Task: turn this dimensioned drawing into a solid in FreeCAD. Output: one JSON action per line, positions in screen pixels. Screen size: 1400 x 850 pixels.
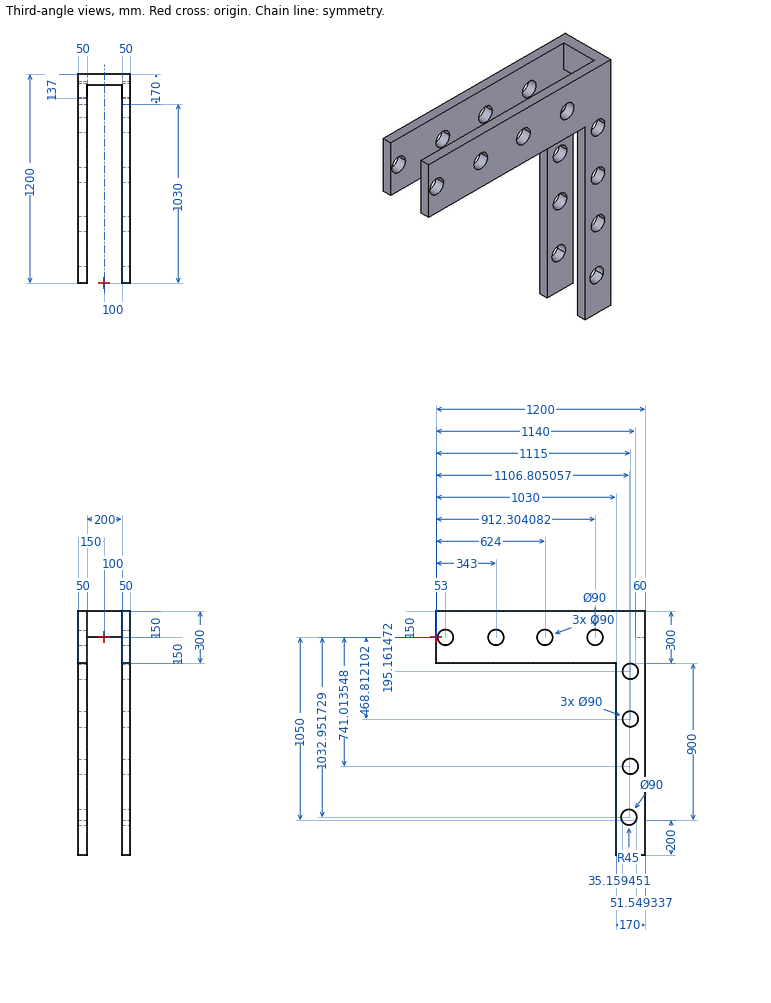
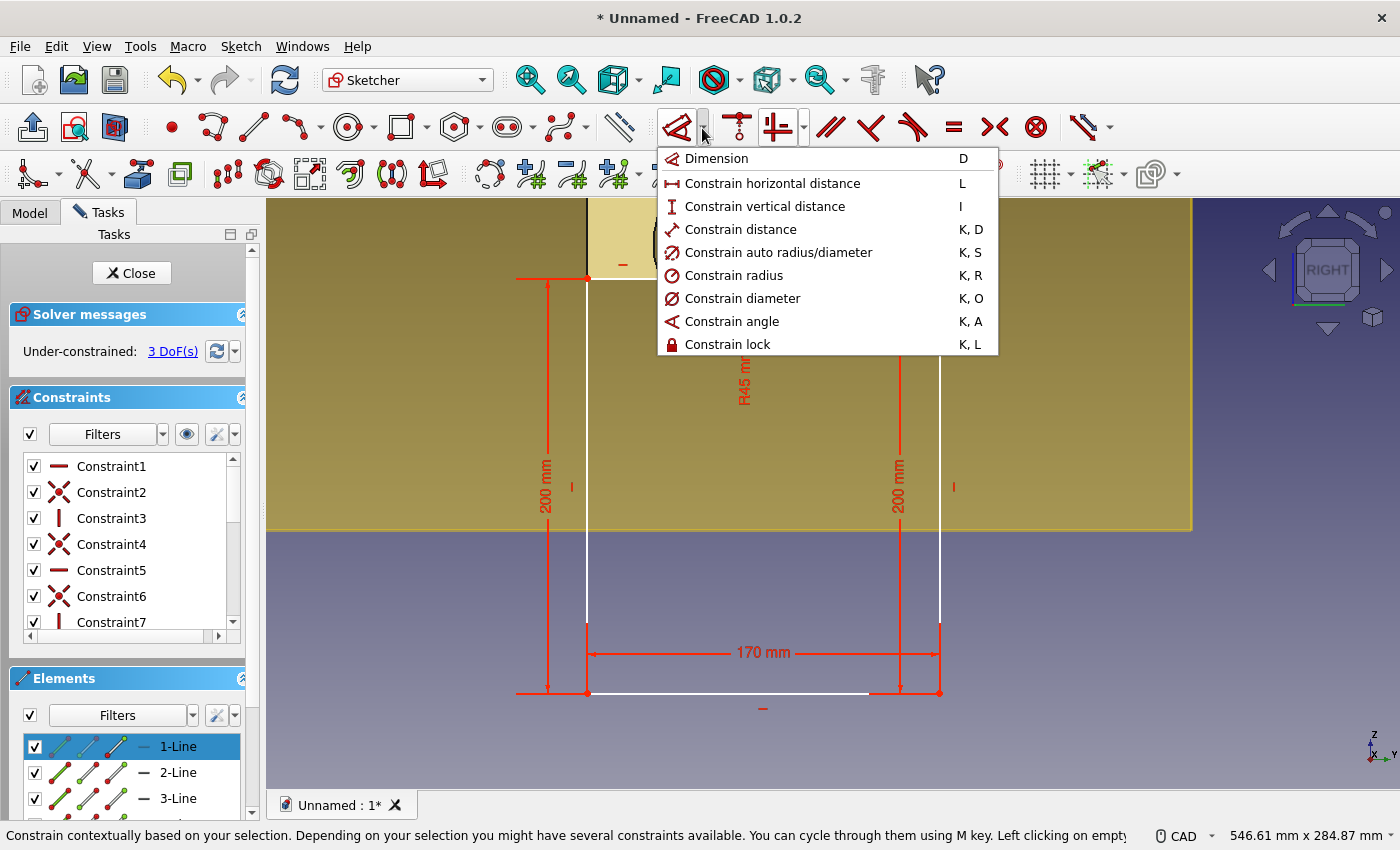
{"action": "left_click", "coordinate": [828, 184]}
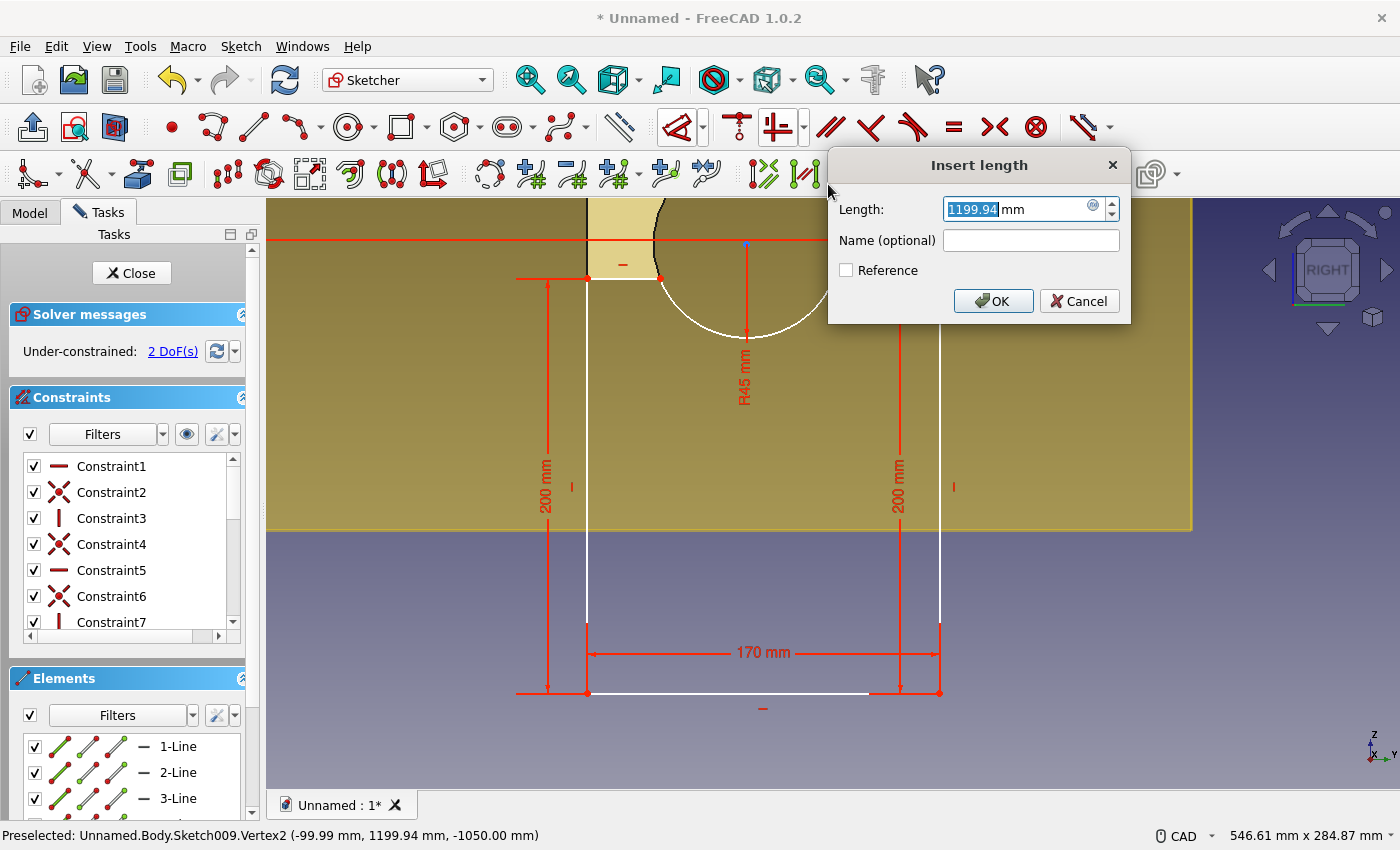
{"action": "type", "text": "1200"}
{"action": "key", "text": "Return"}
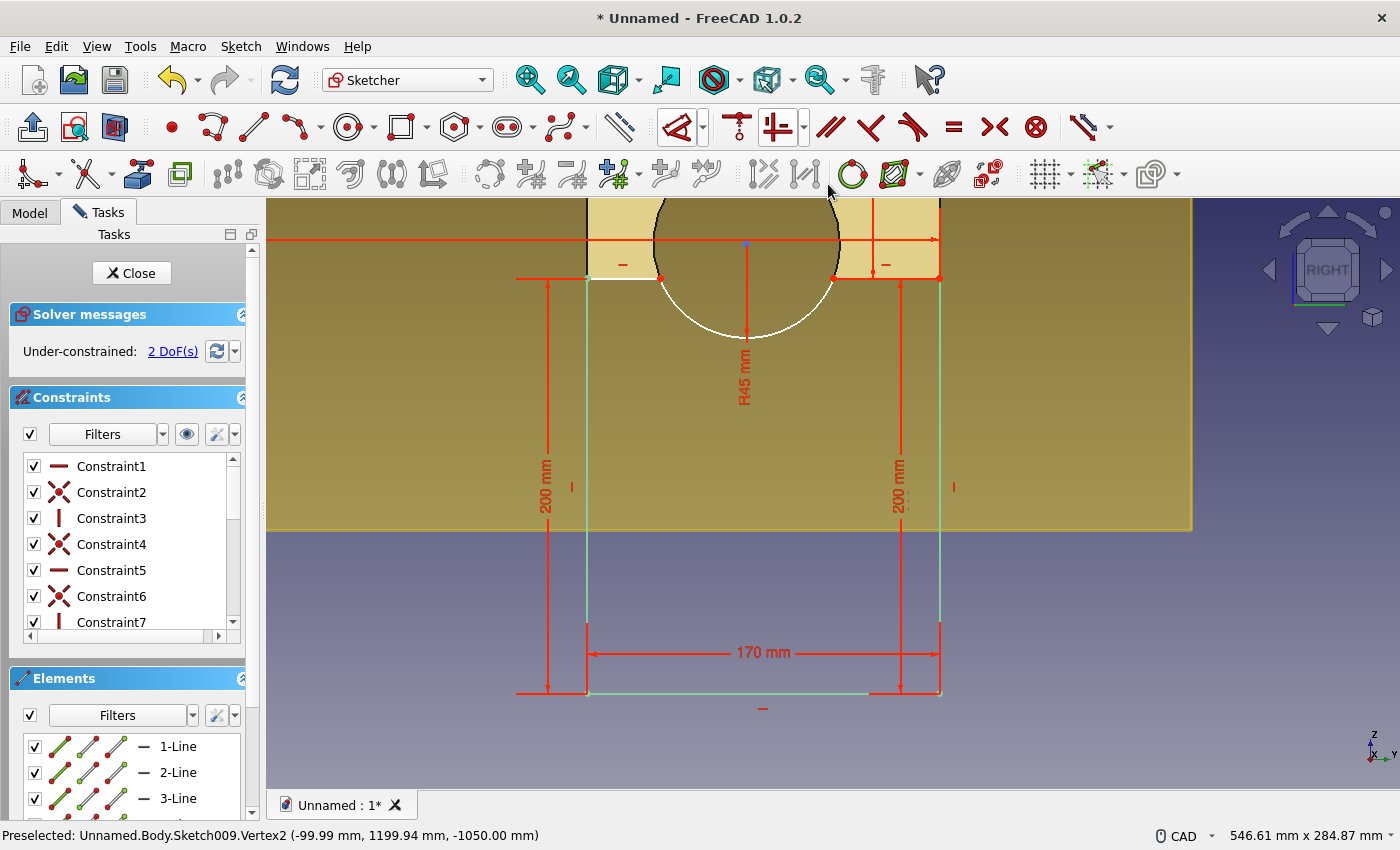
{"action": "left_click", "coordinate": [865, 279]}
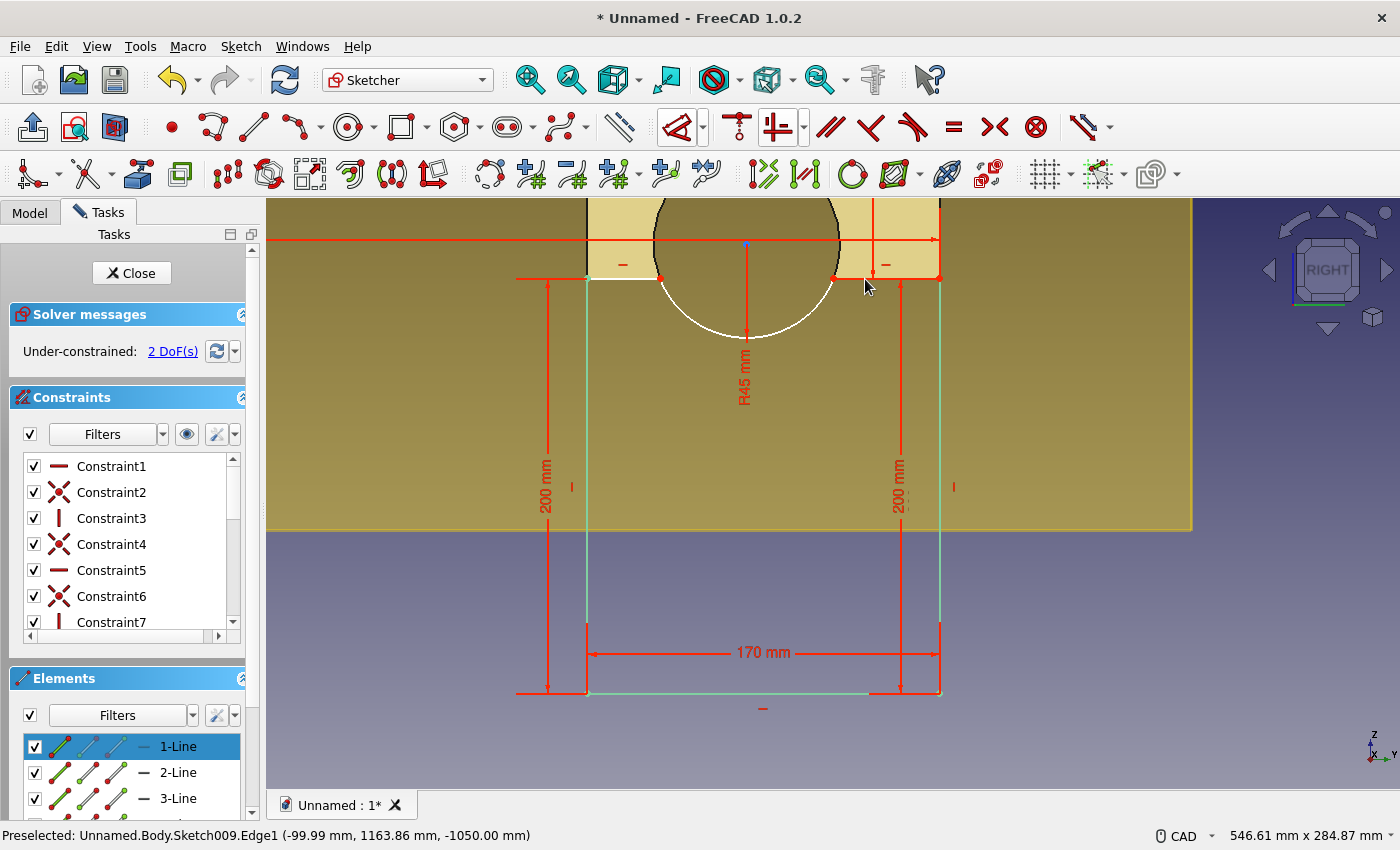
{"action": "key", "text": "l"}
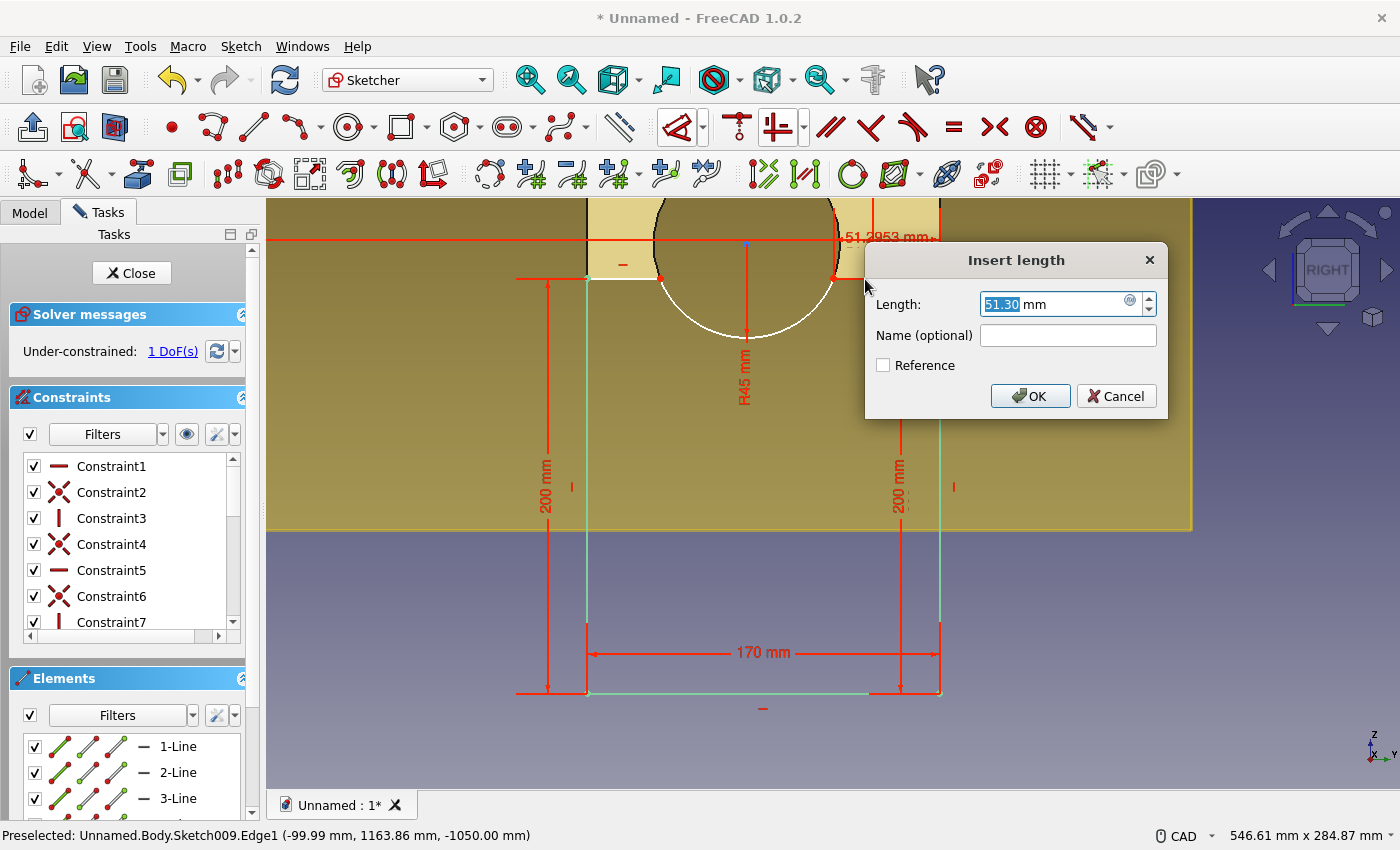
{"action": "type", "text": "51.549337"}
{"action": "key", "text": "Return"}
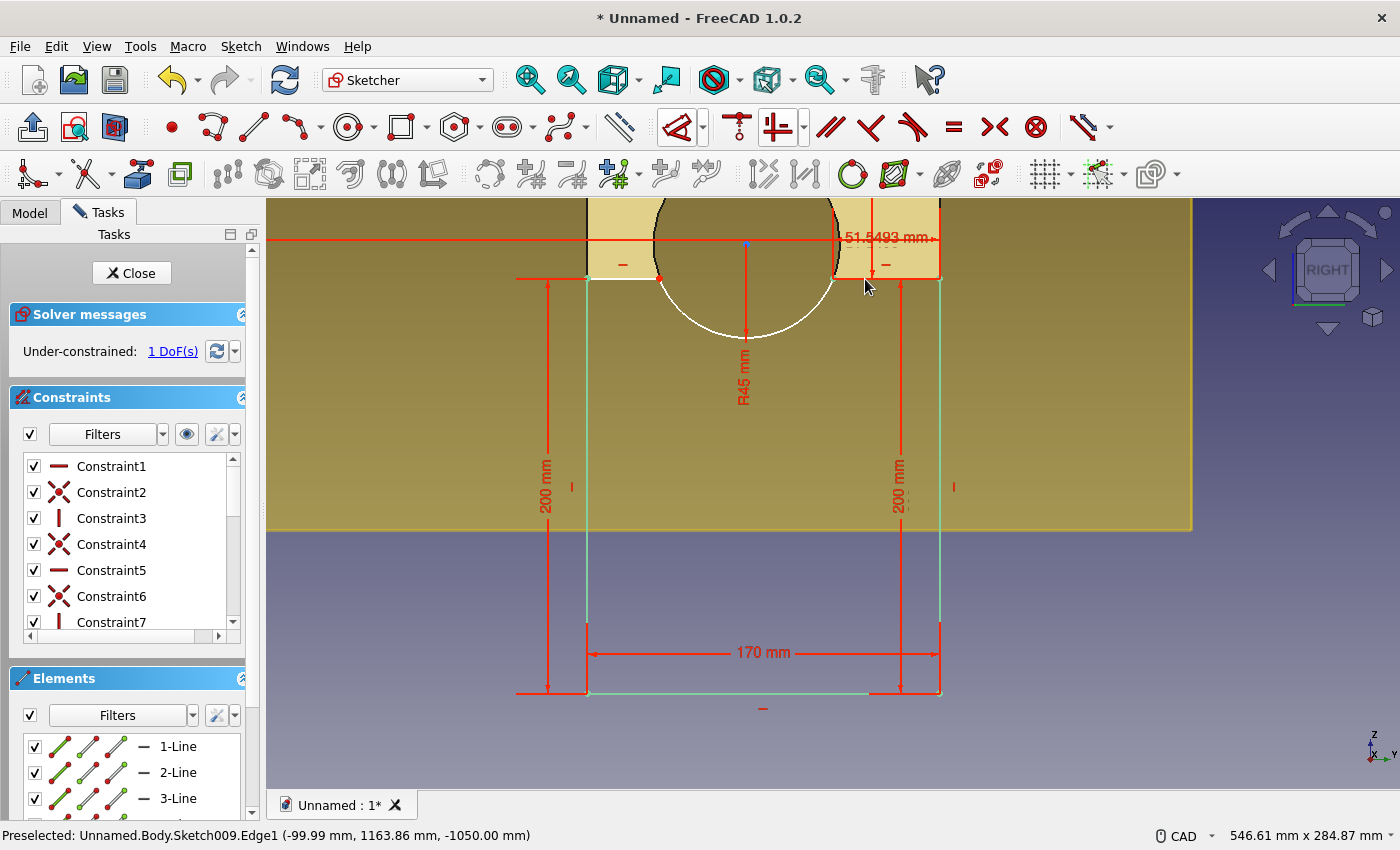
{"action": "left_click", "coordinate": [609, 279]}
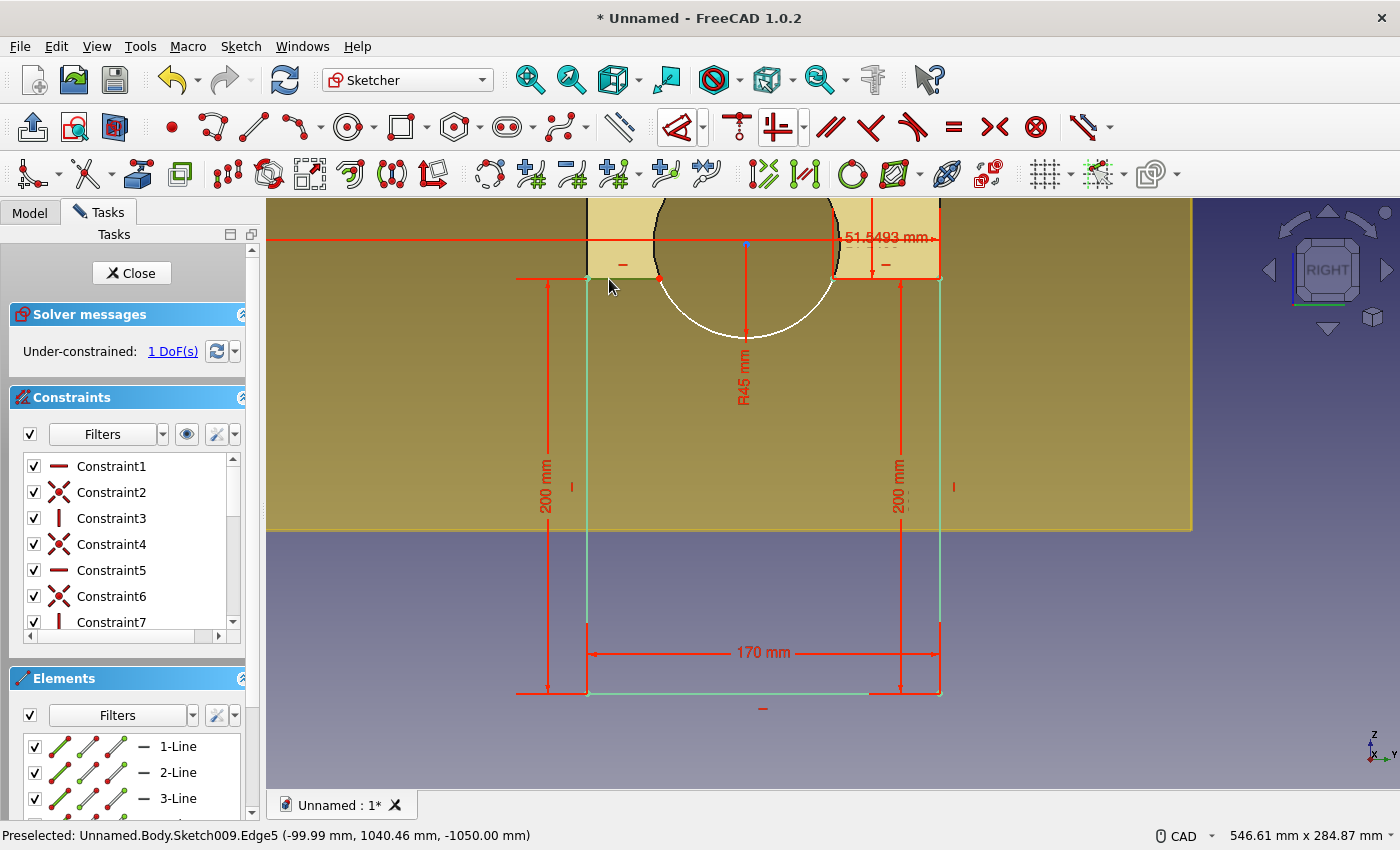
{"action": "left_click", "coordinate": [702, 128]}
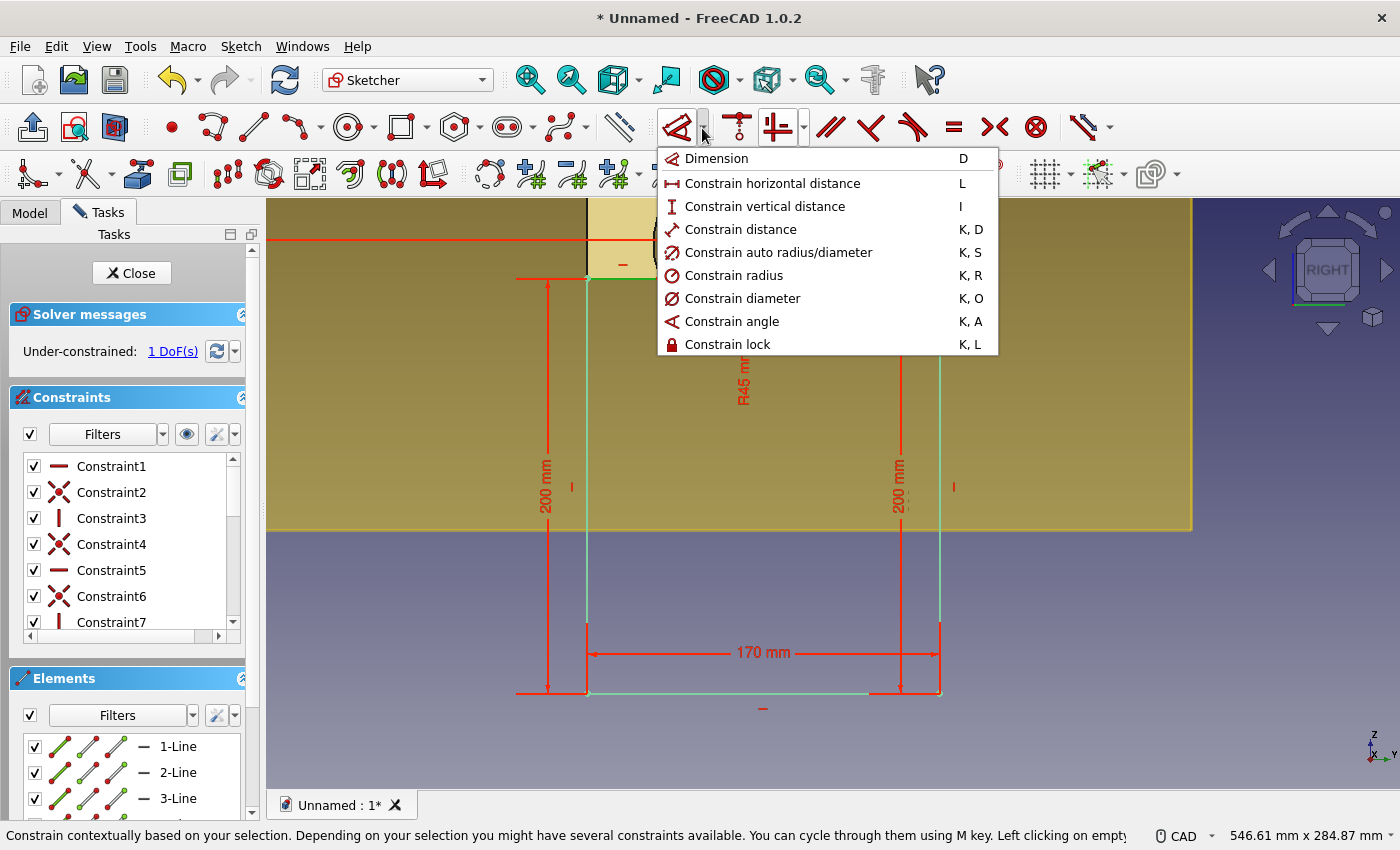
{"action": "left_click", "coordinate": [828, 184]}